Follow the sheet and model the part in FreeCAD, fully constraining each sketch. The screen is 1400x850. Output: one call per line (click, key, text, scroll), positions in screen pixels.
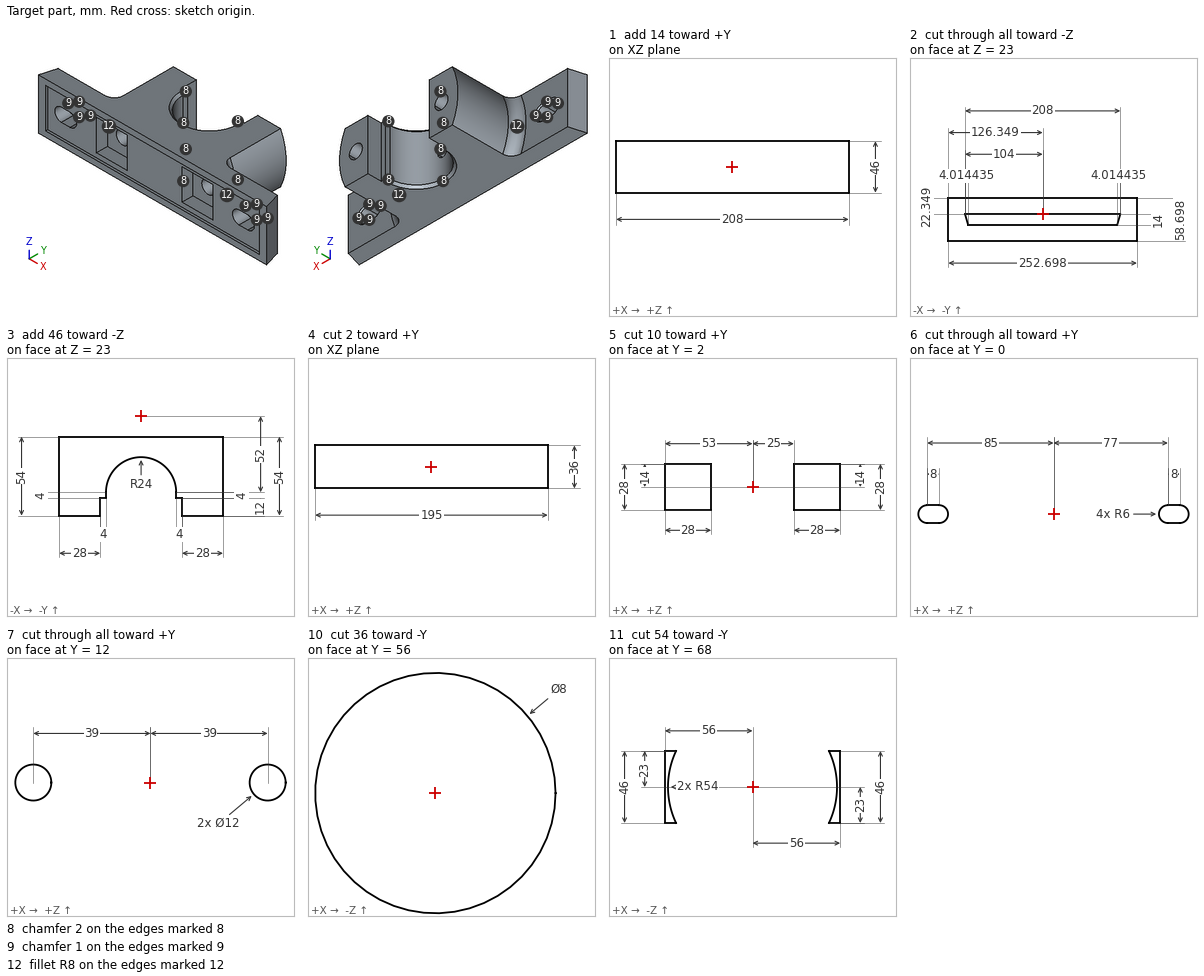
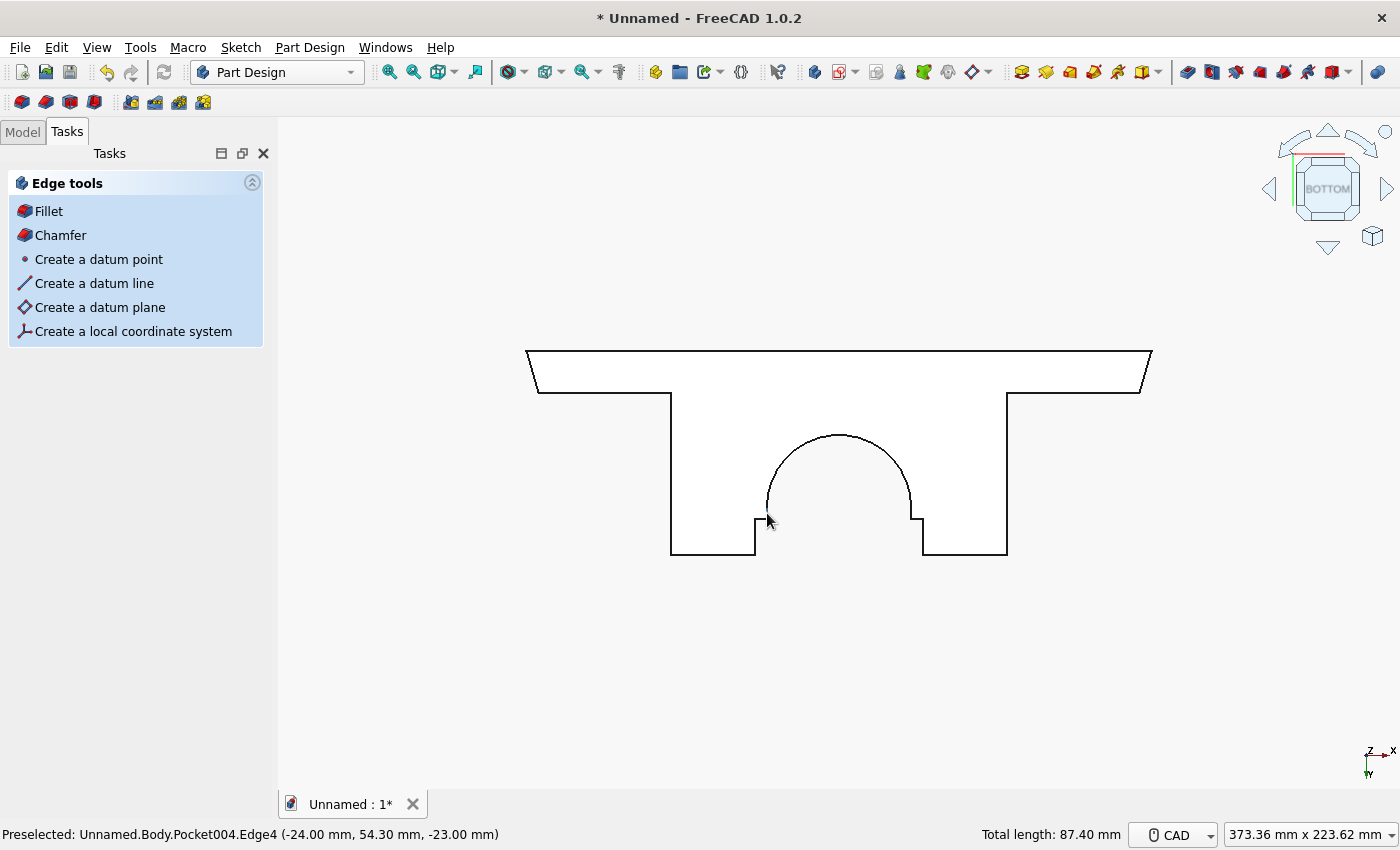
click(911, 513, ctrl)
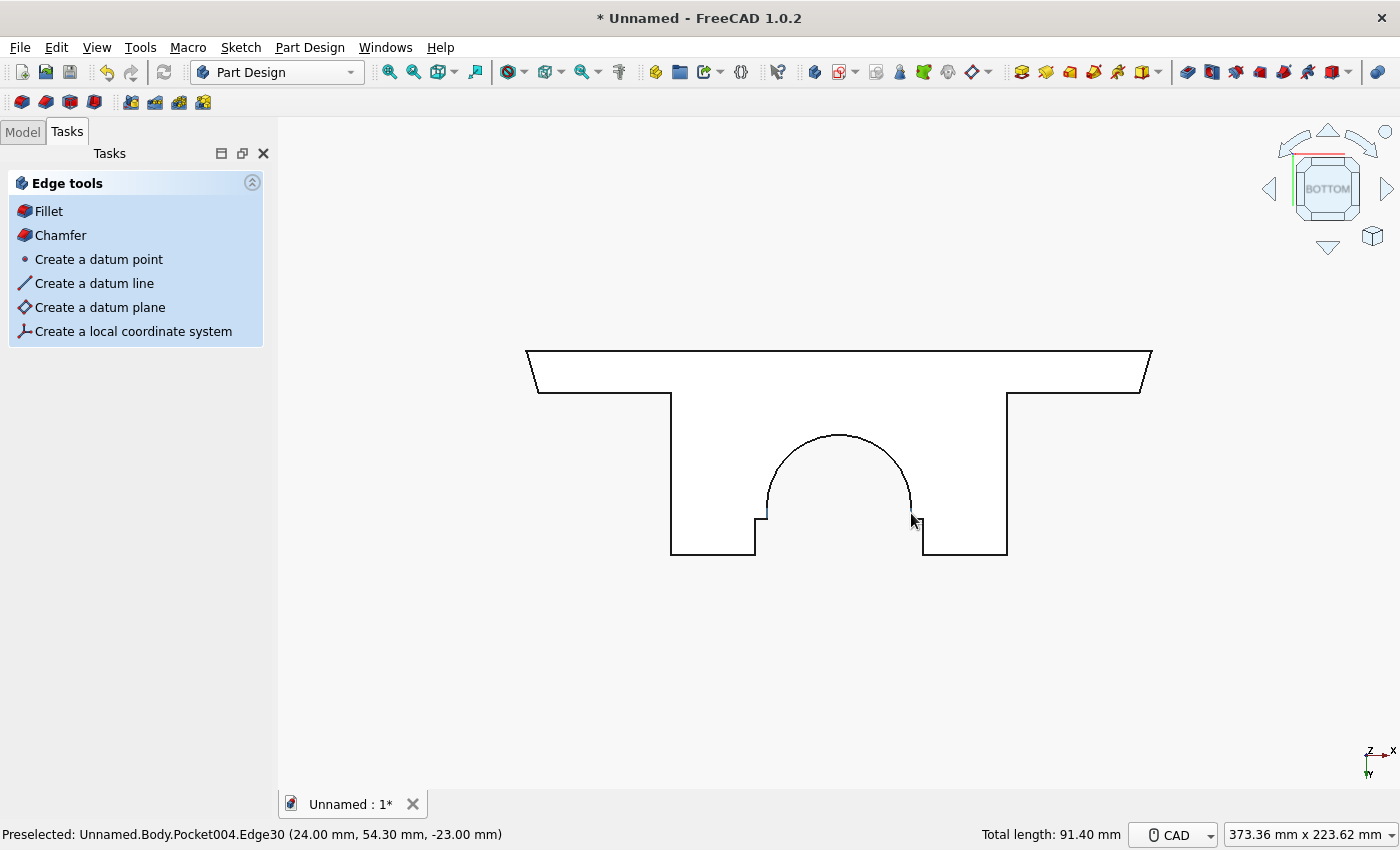
key(4)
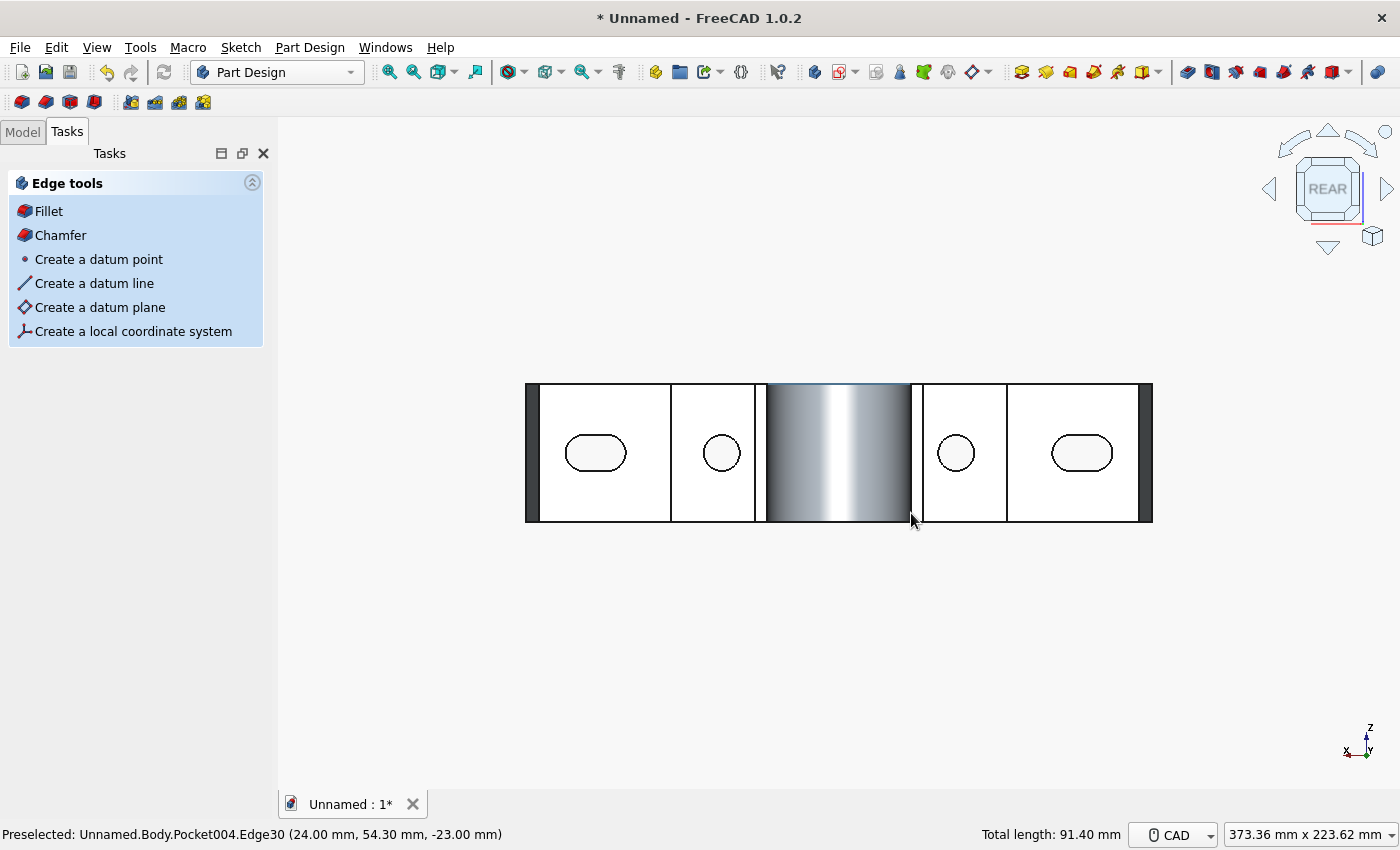
click(839, 521, ctrl)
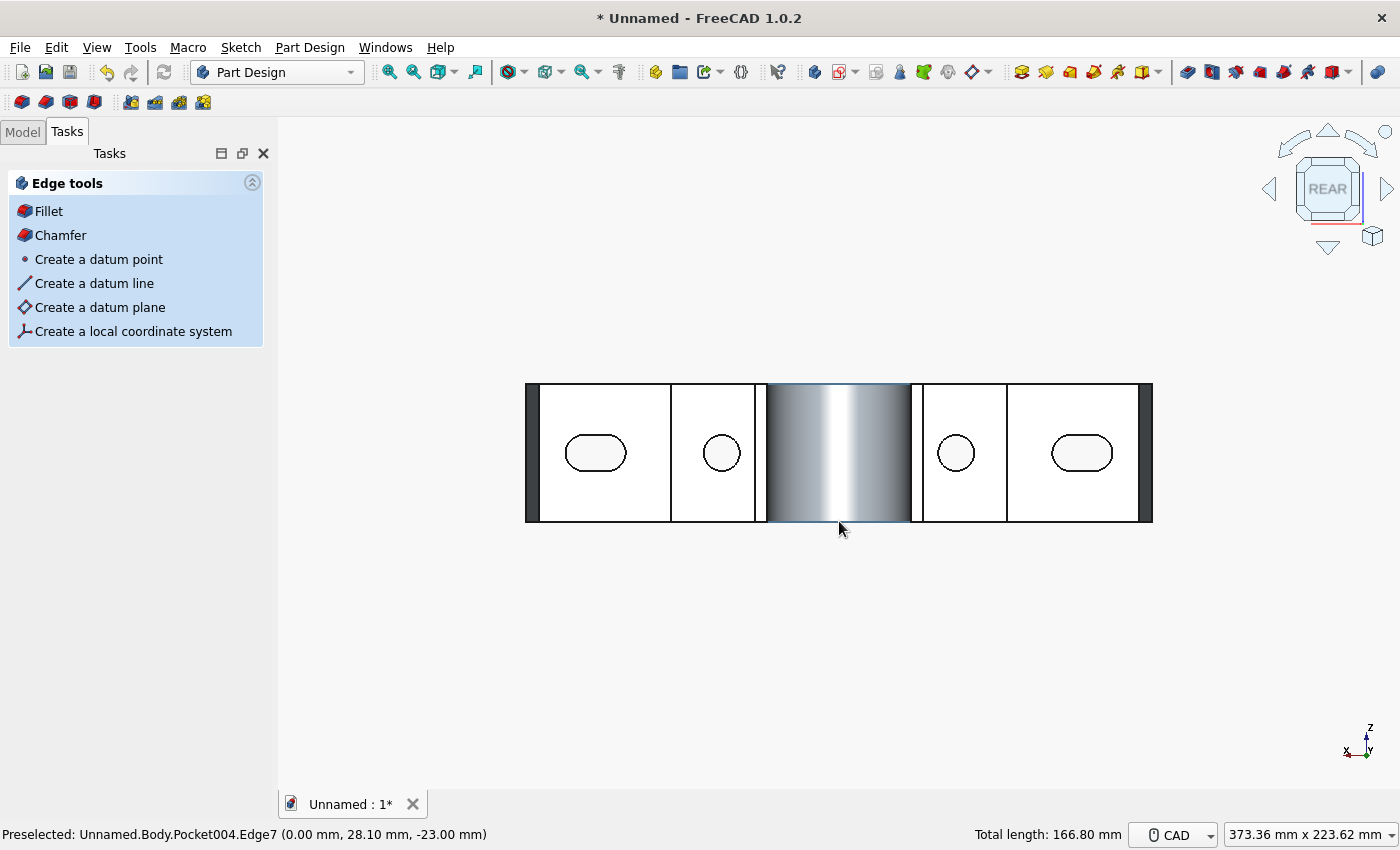
click(46, 102)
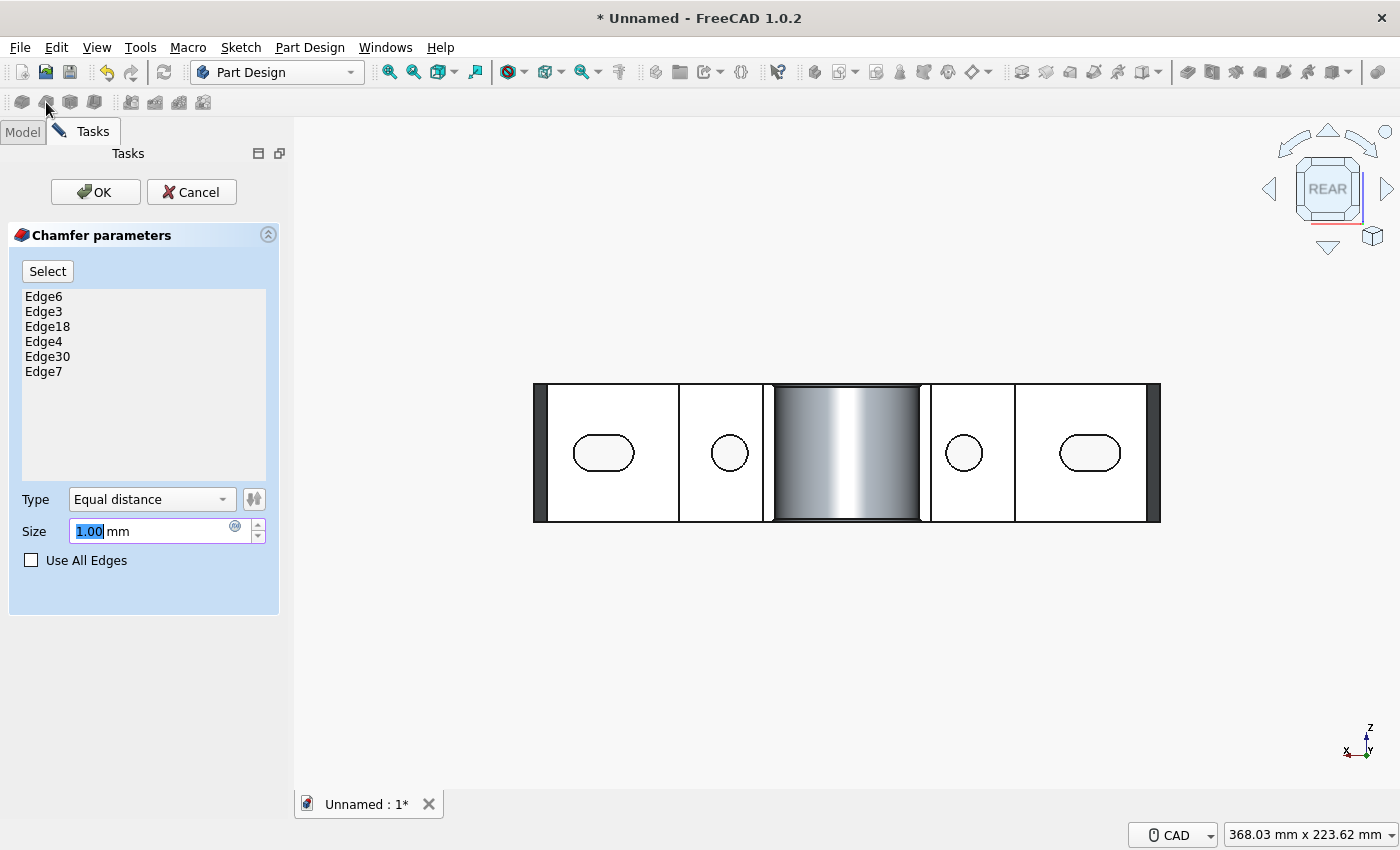
text(2)
key(Tab)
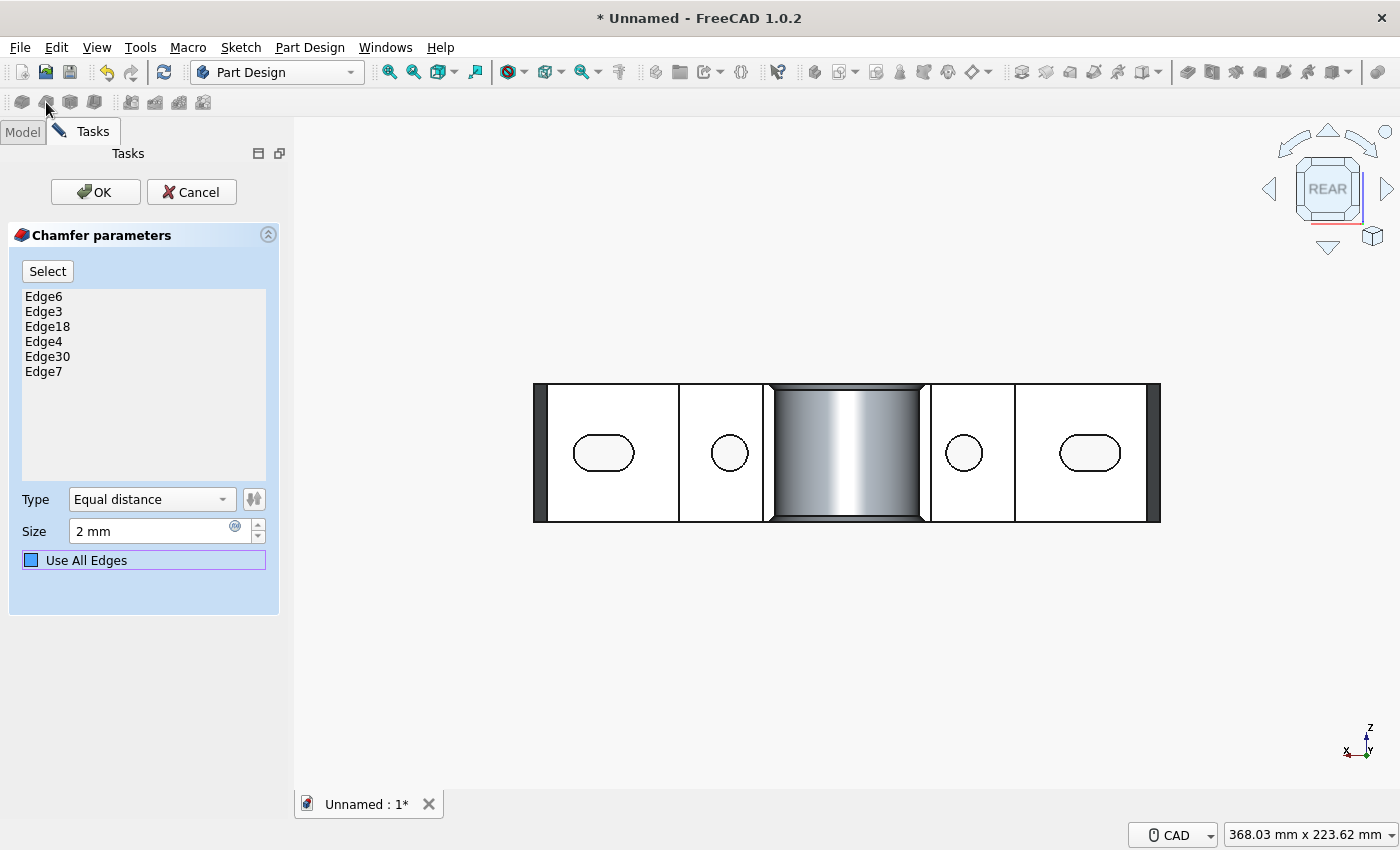
click(96, 192)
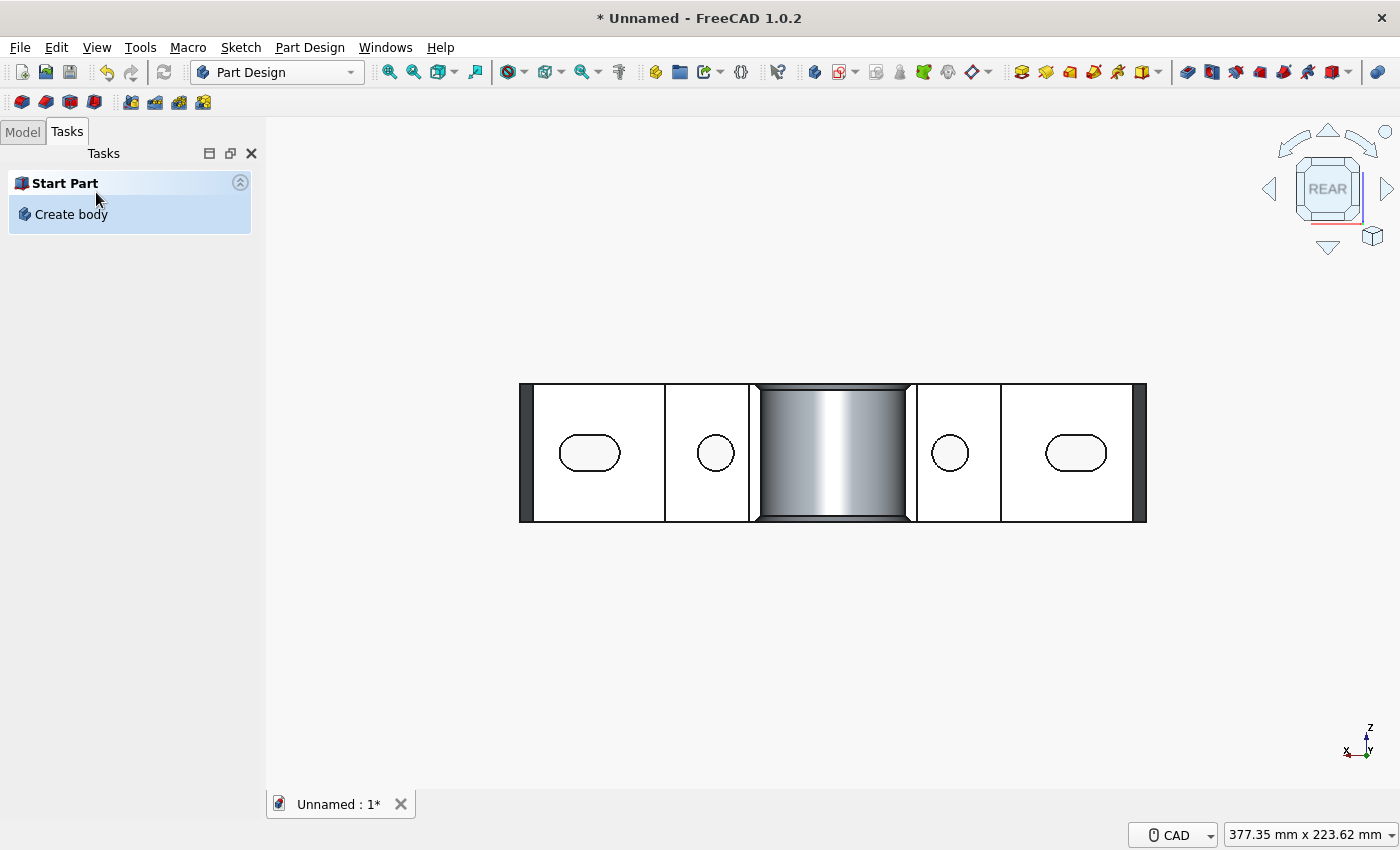
click(620, 452)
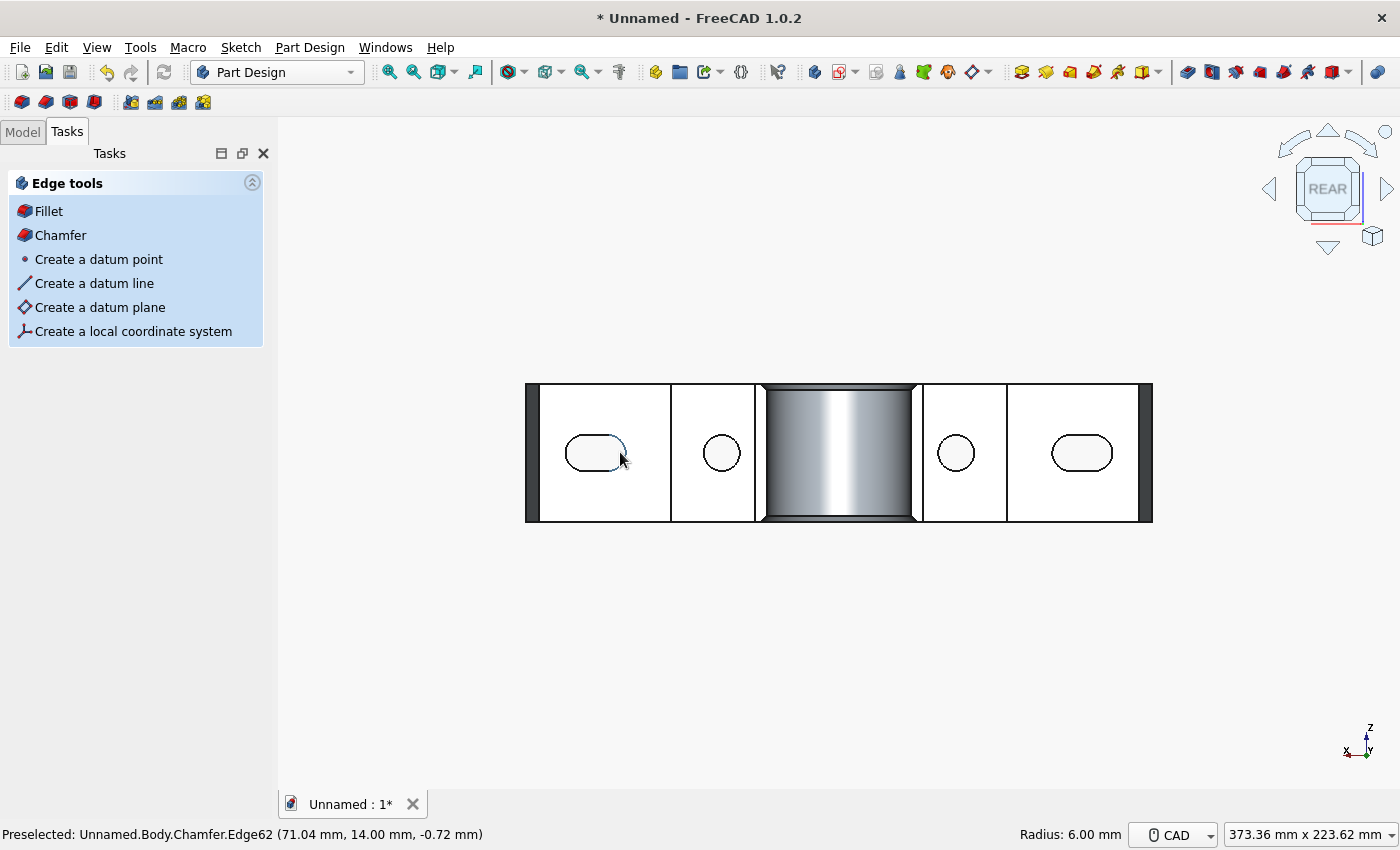
click(596, 434, ctrl)